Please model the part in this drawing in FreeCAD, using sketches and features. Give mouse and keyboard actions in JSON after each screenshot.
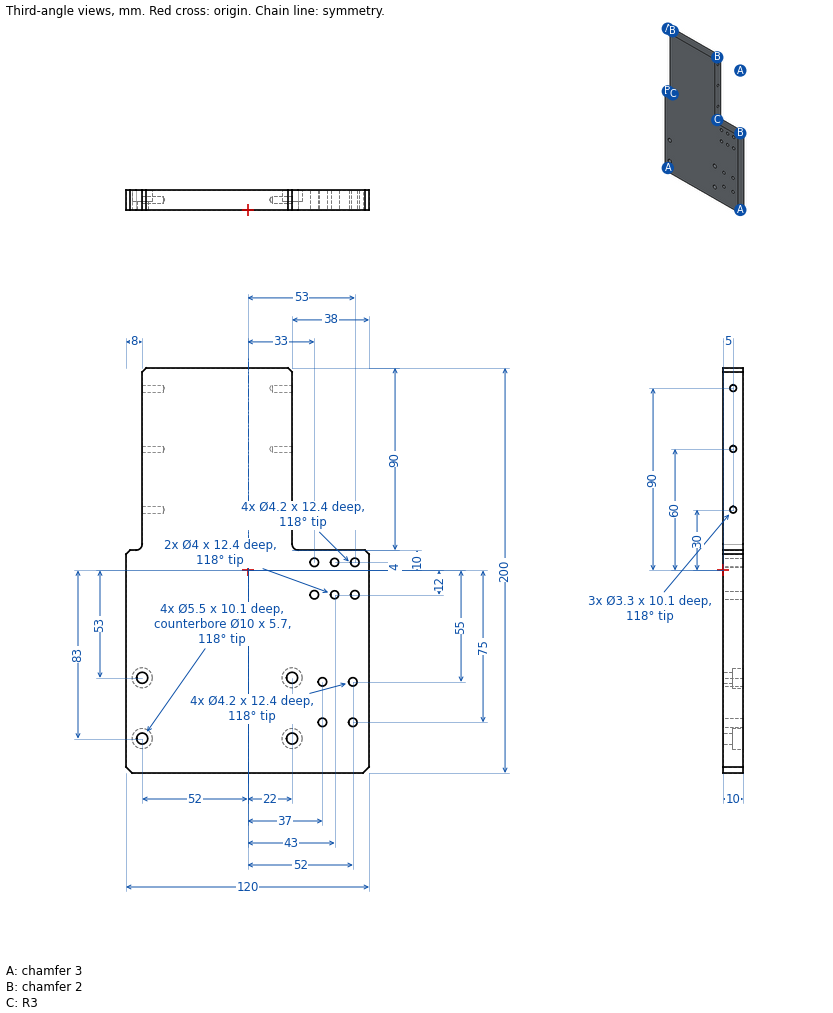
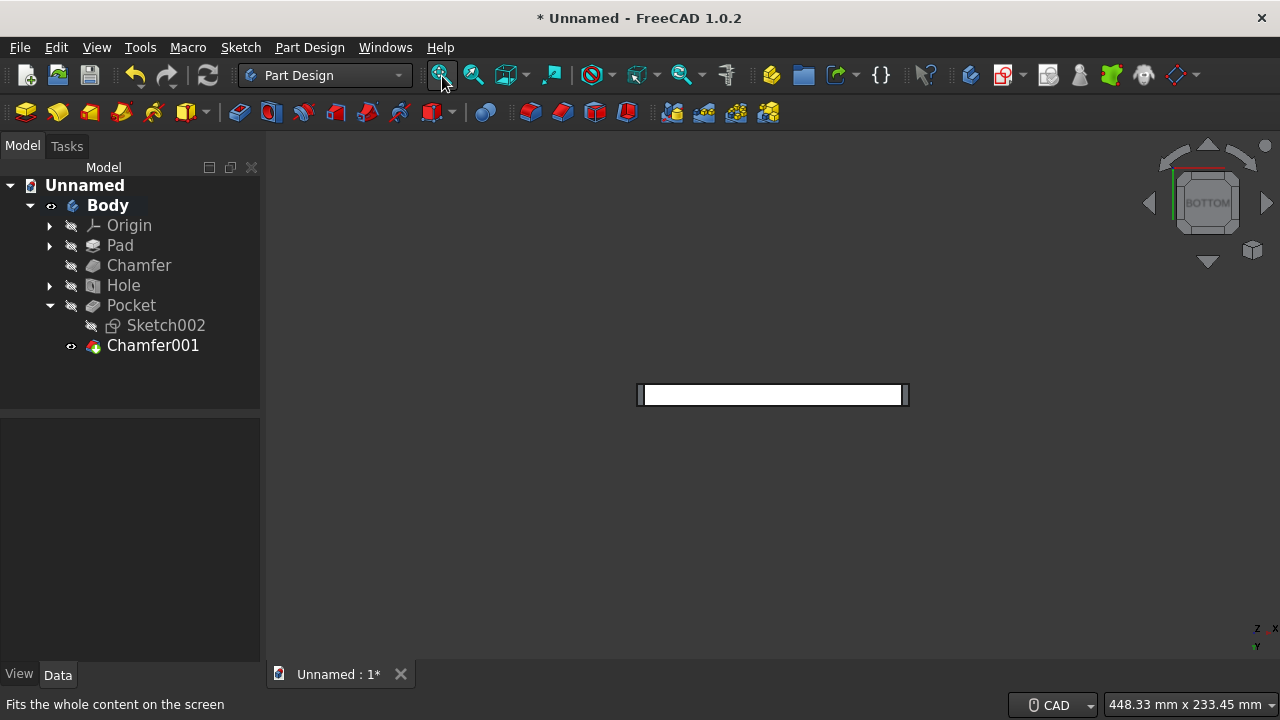
{"action": "left_click", "coordinate": [442, 76]}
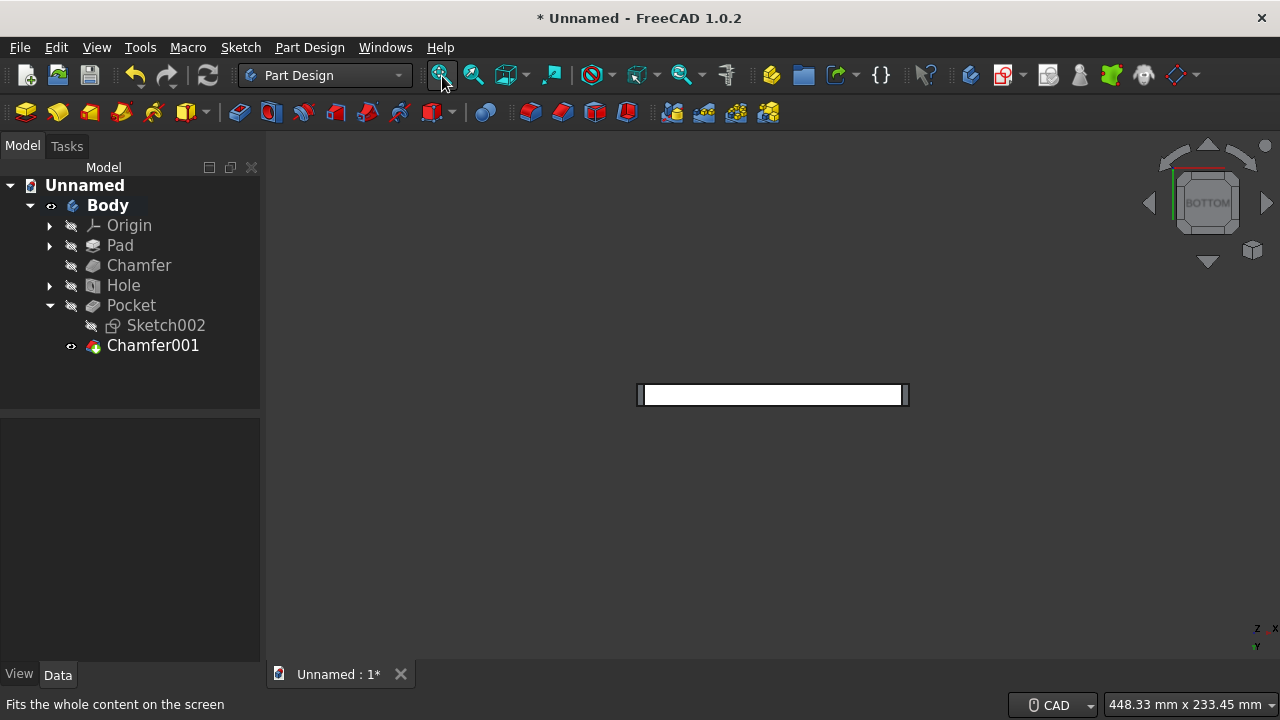
{"action": "key", "text": "4"}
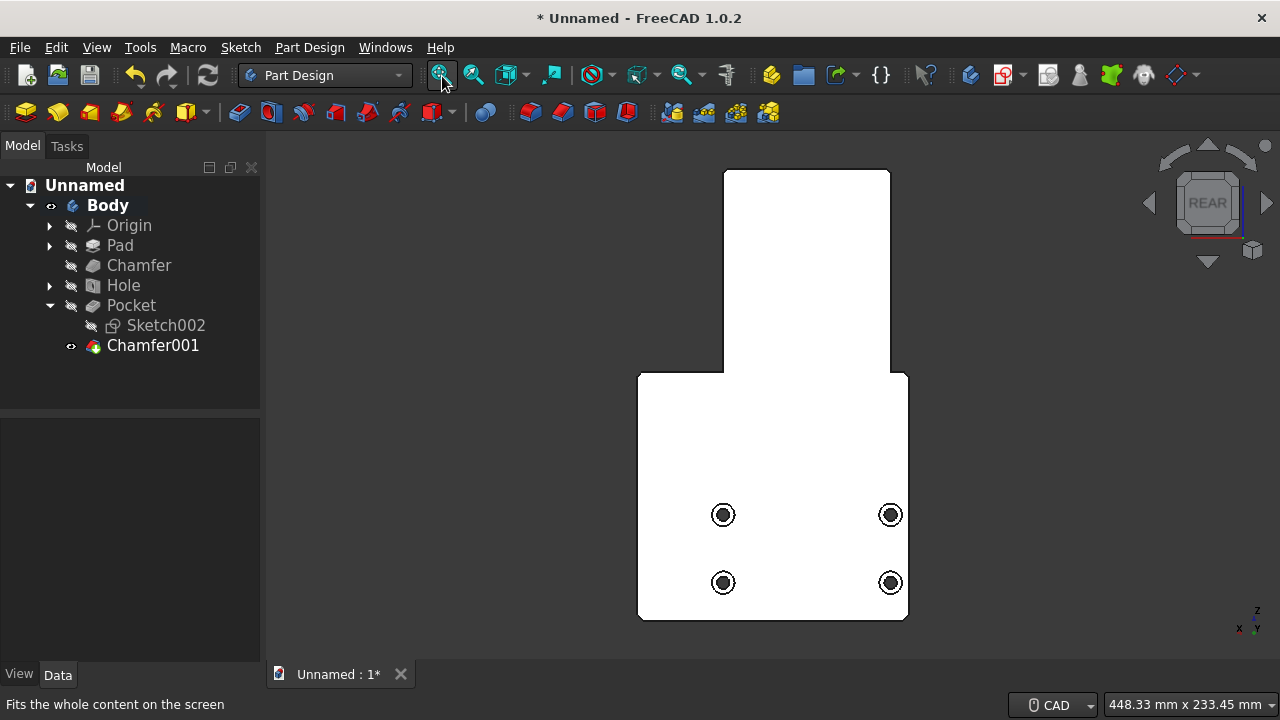
{"action": "key", "text": "6"}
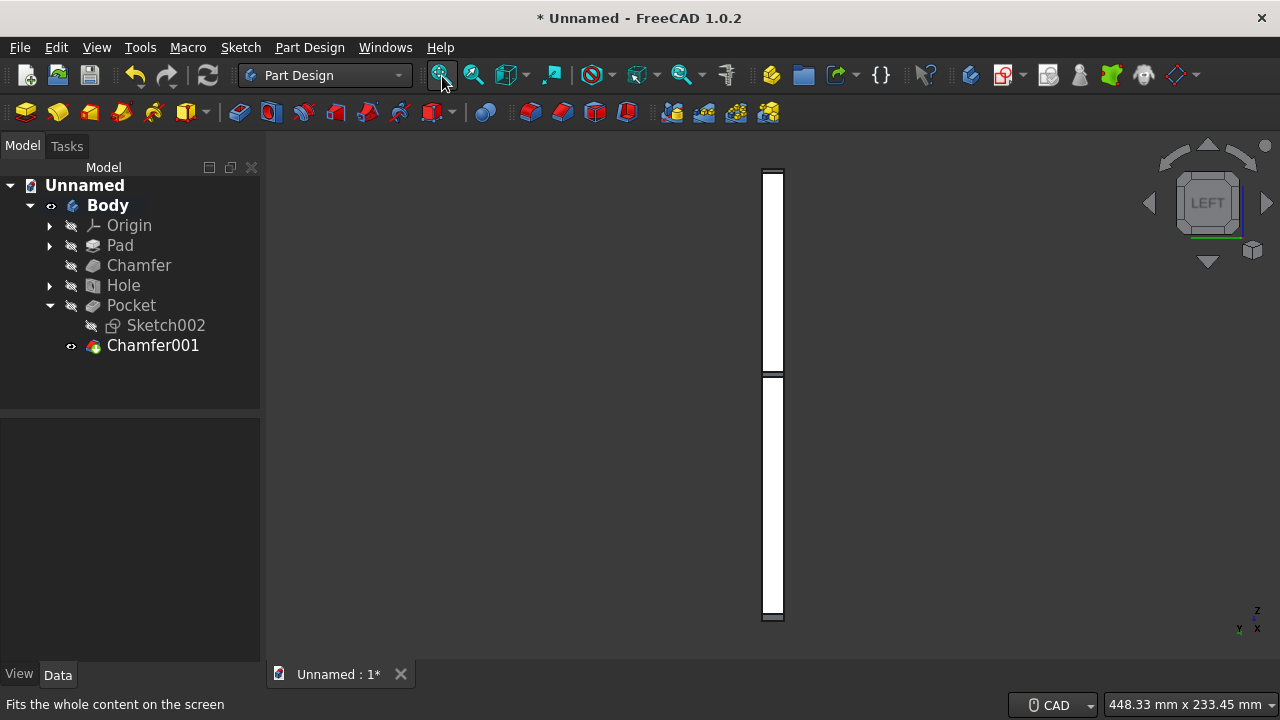
{"action": "key", "text": "v 3"}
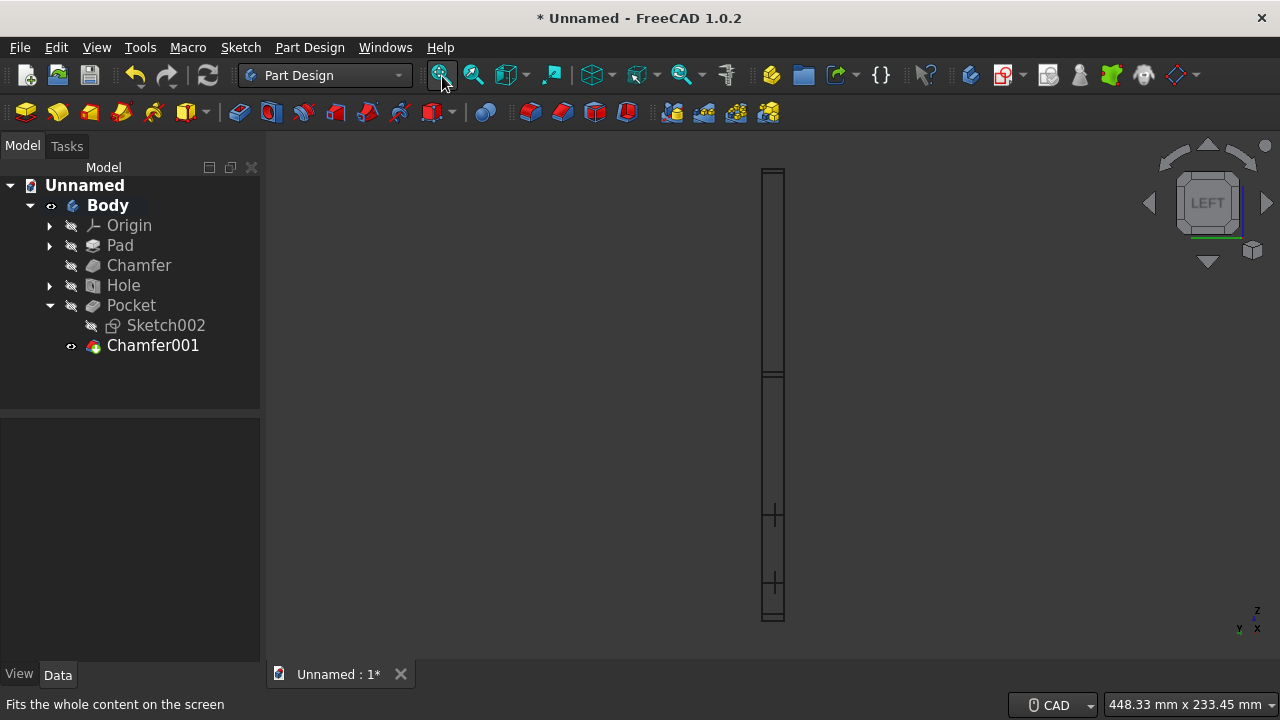
{"action": "key", "text": "0"}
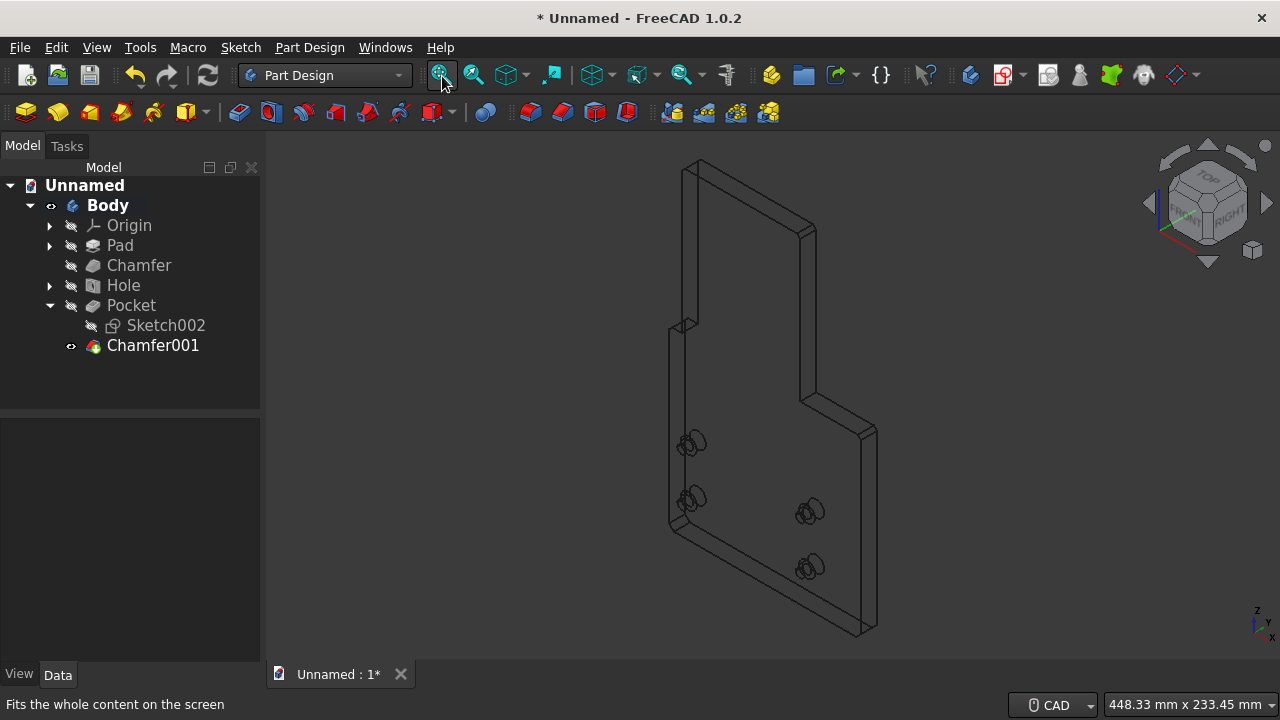
{"action": "left_click", "coordinate": [808, 396]}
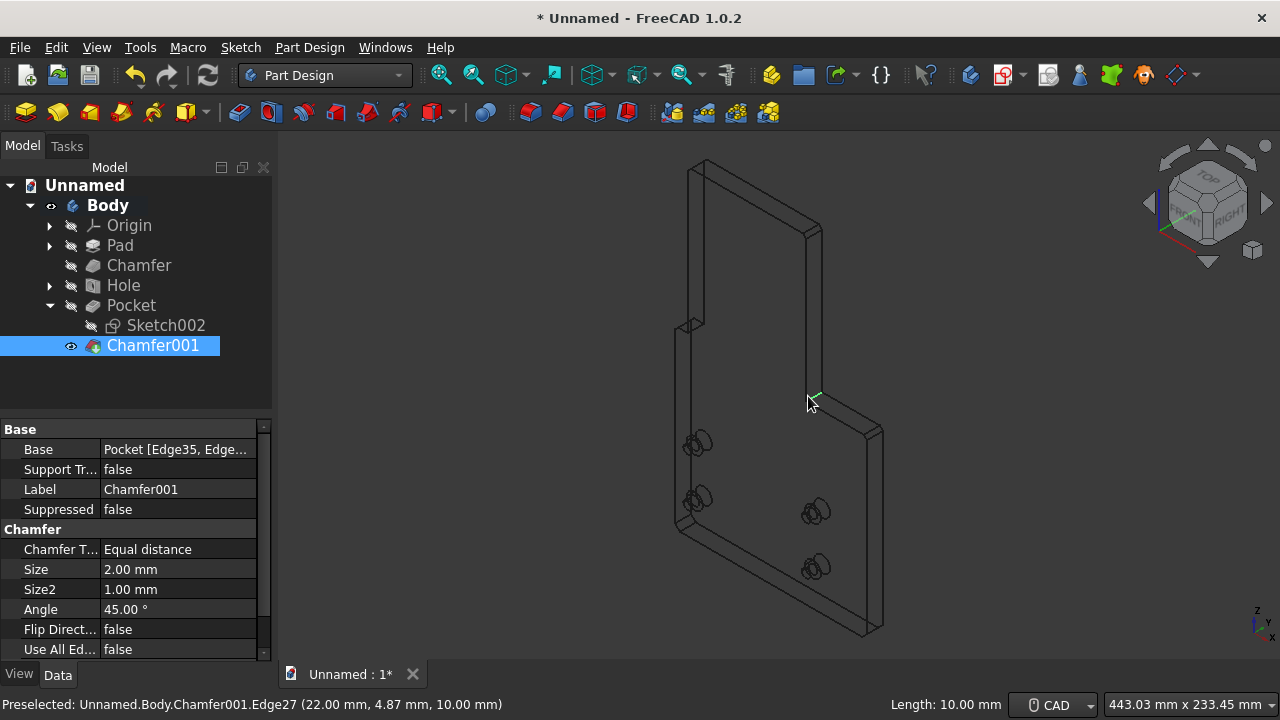
{"action": "left_click", "coordinate": [696, 328], "text": "ctrl"}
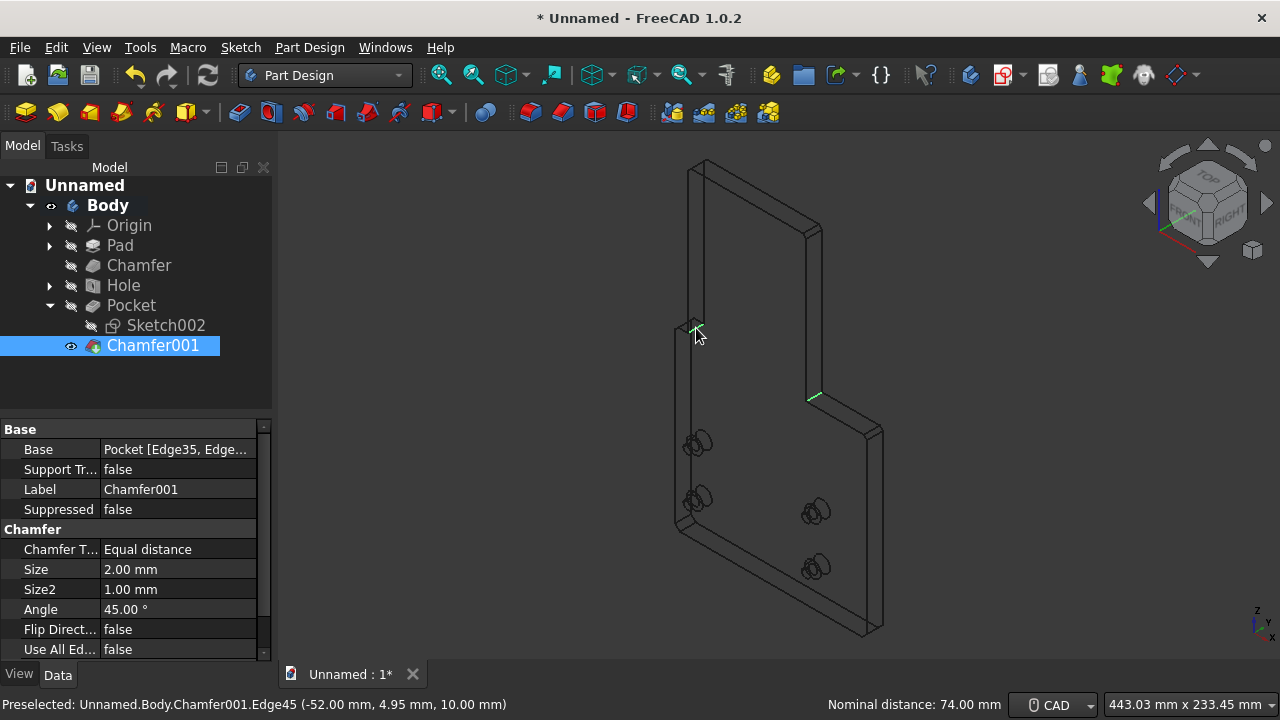
{"action": "key", "text": "v 1"}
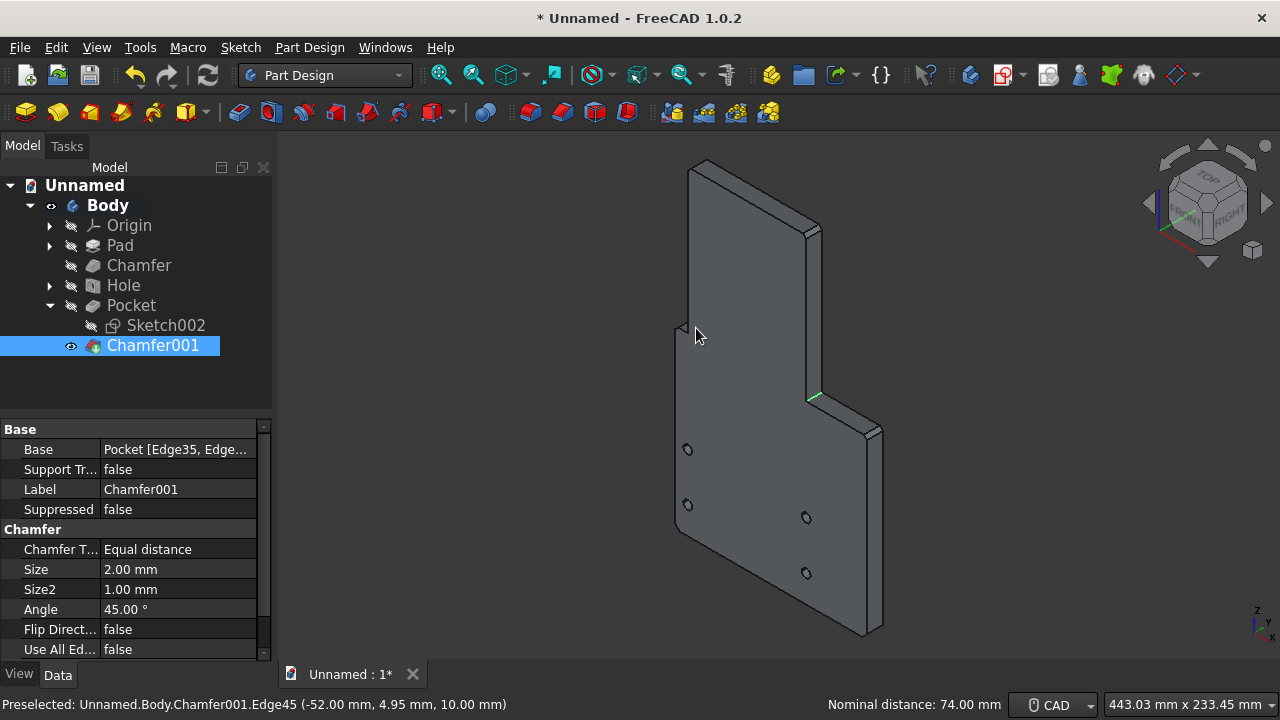
{"action": "left_click", "coordinate": [532, 112]}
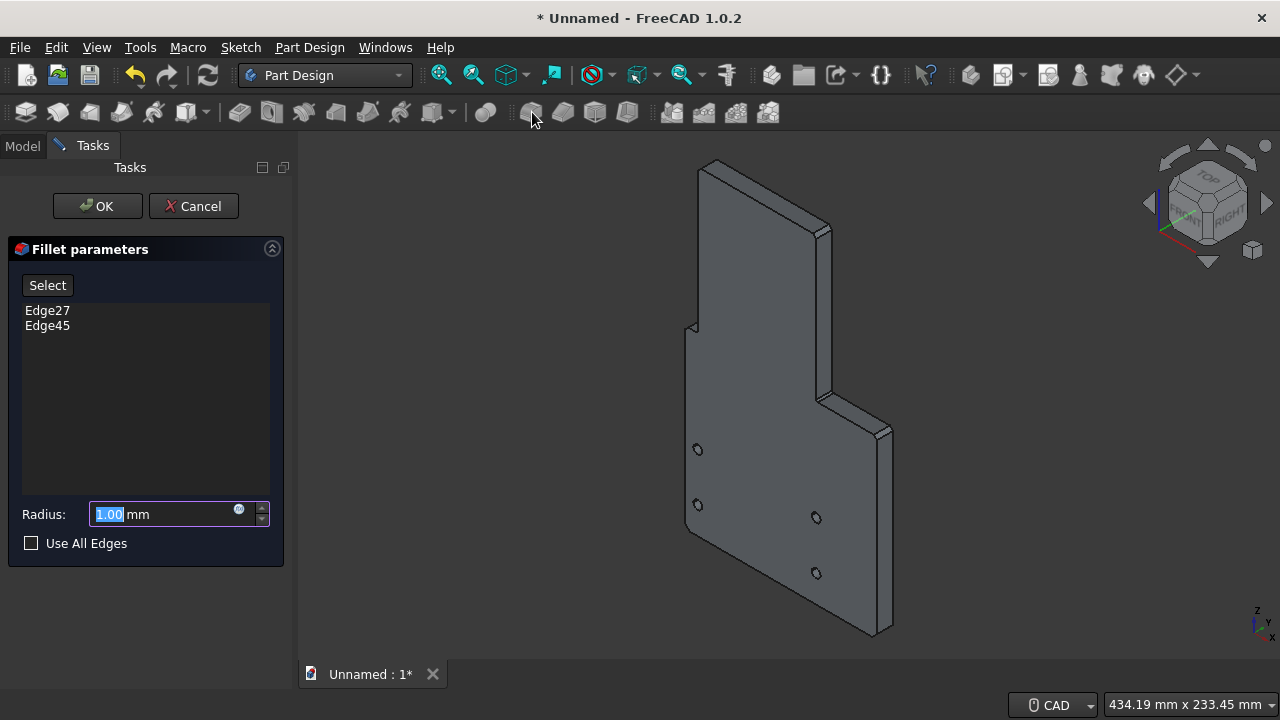
{"action": "type", "text": "3"}
{"action": "key", "text": "Tab"}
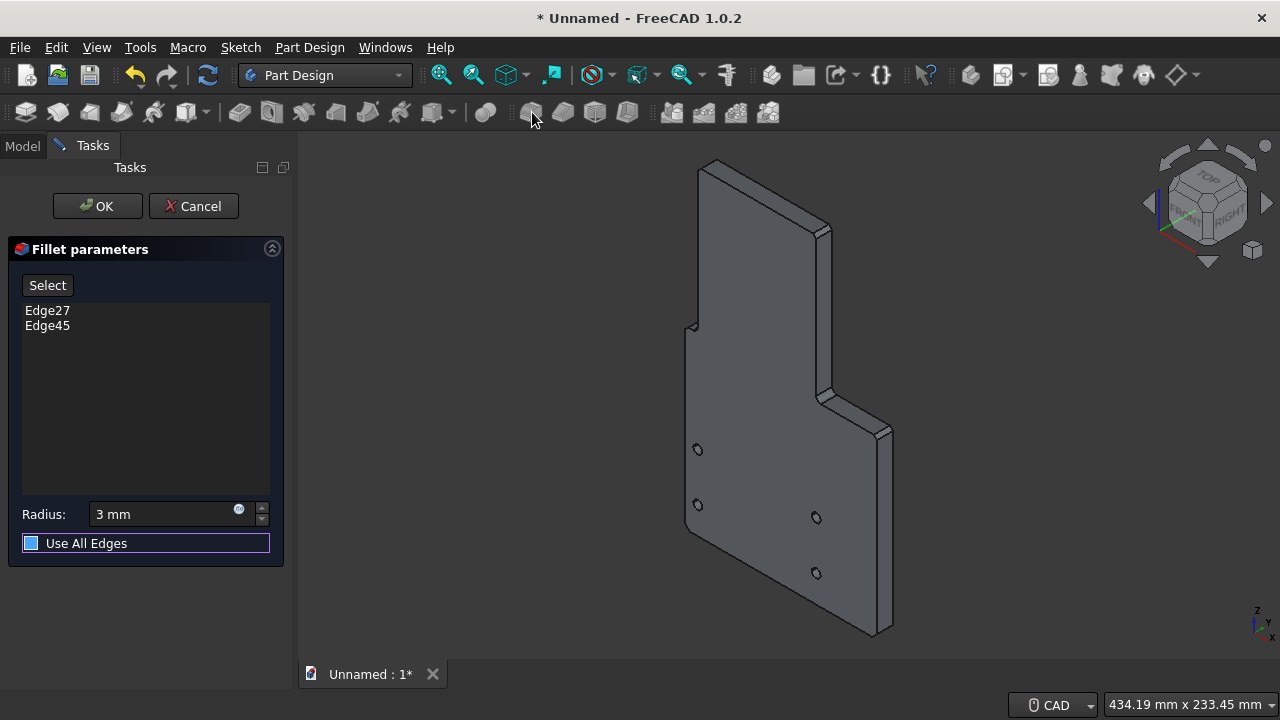
{"action": "left_click", "coordinate": [98, 206]}